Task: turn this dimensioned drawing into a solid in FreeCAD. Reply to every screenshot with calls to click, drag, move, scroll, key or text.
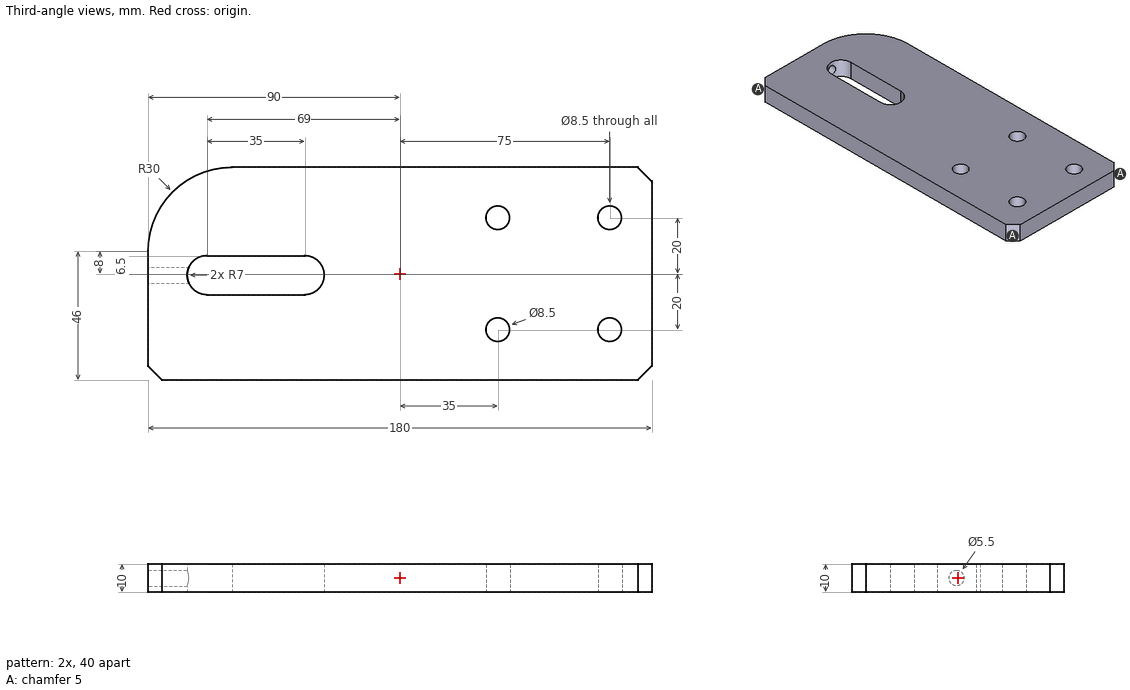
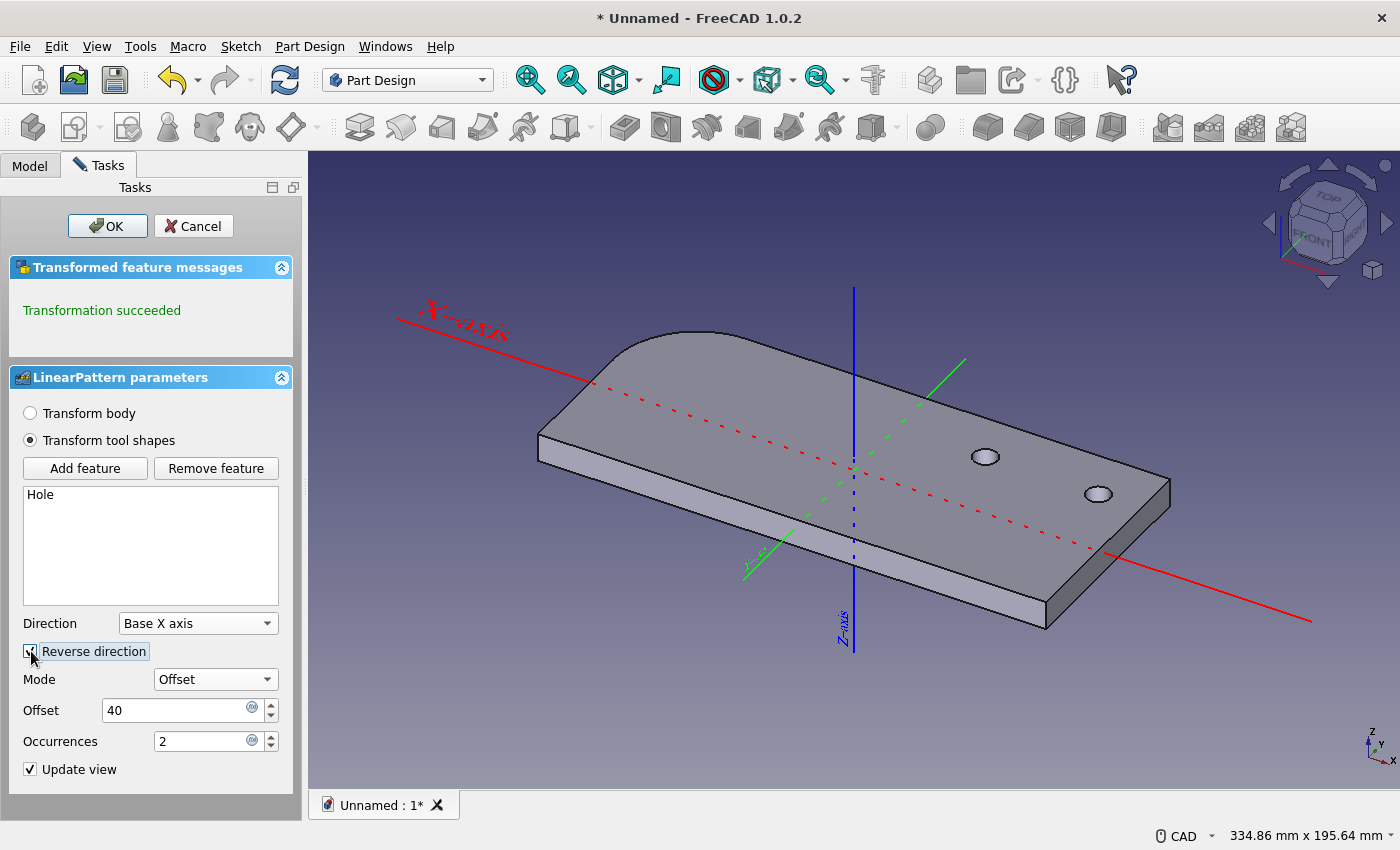
click(108, 226)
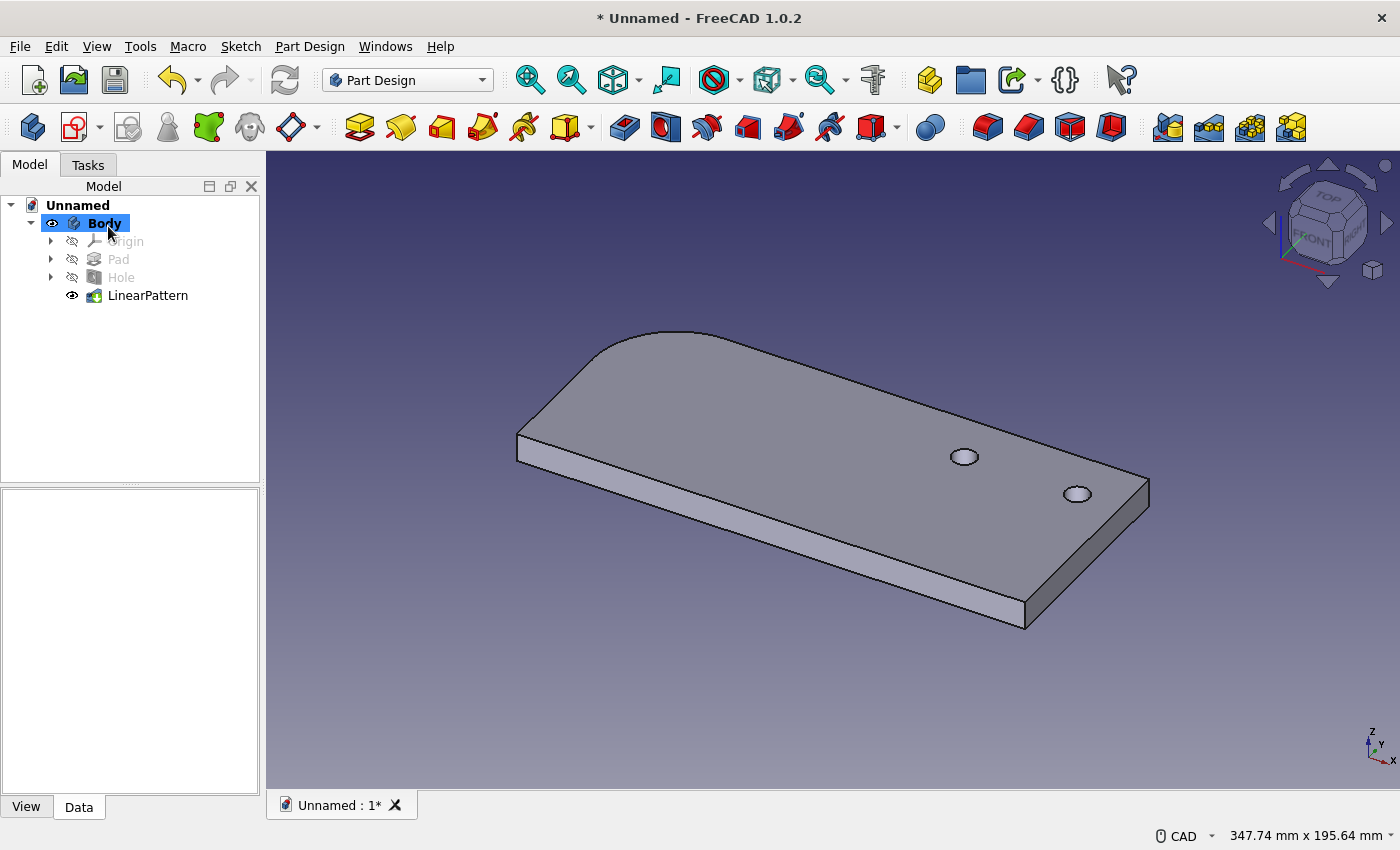
click(117, 277)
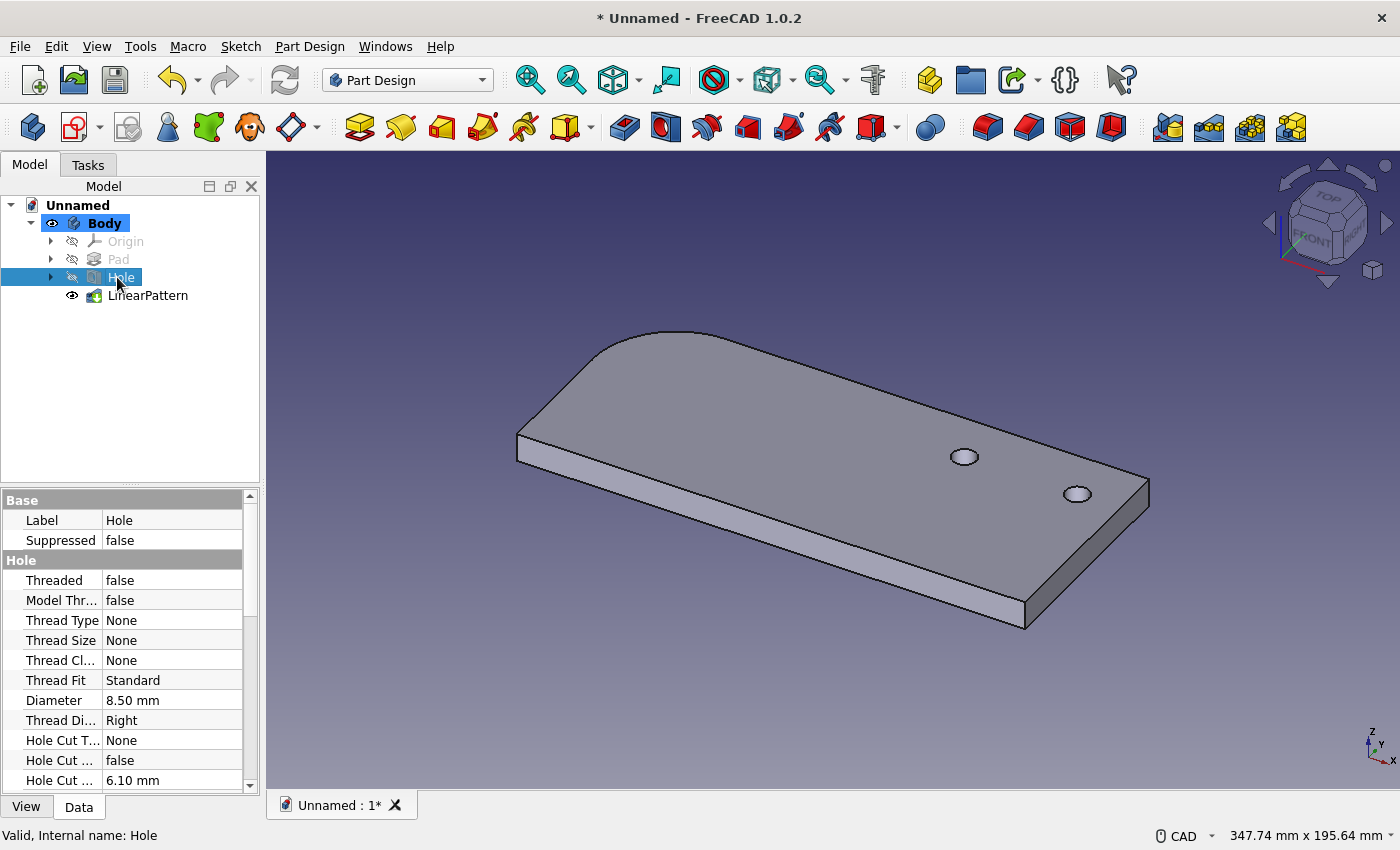
click(1168, 128)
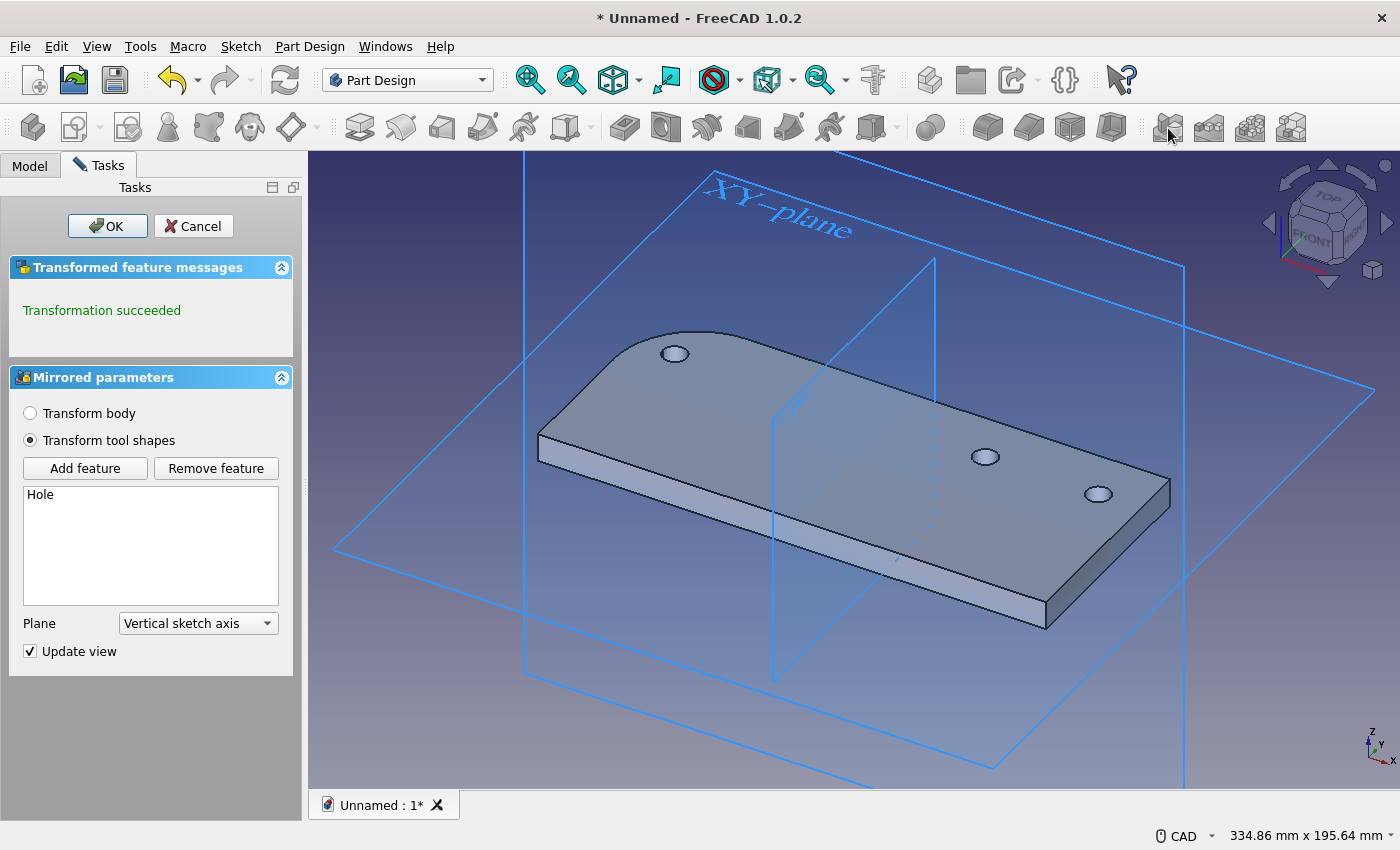
click(199, 624)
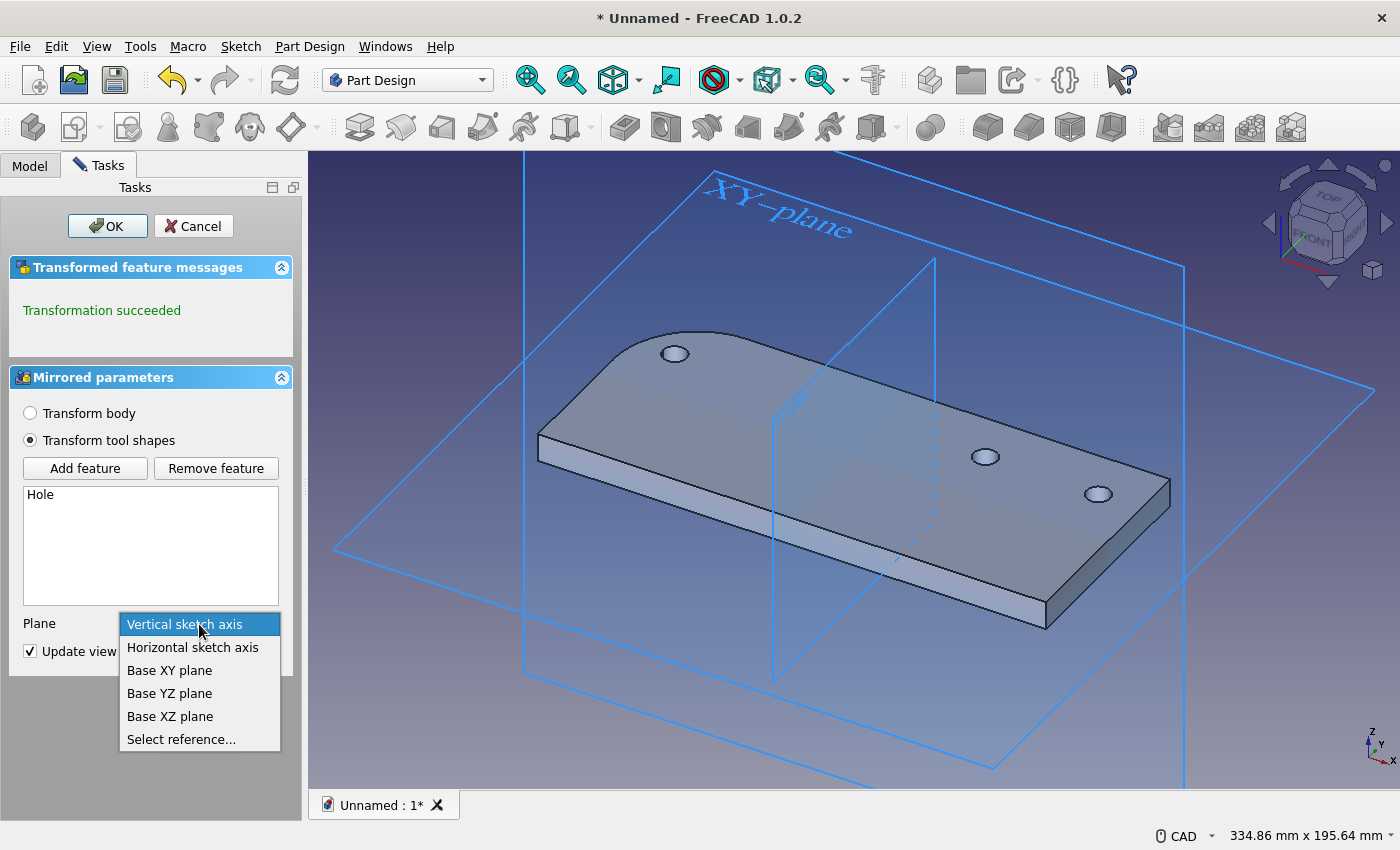
click(198, 716)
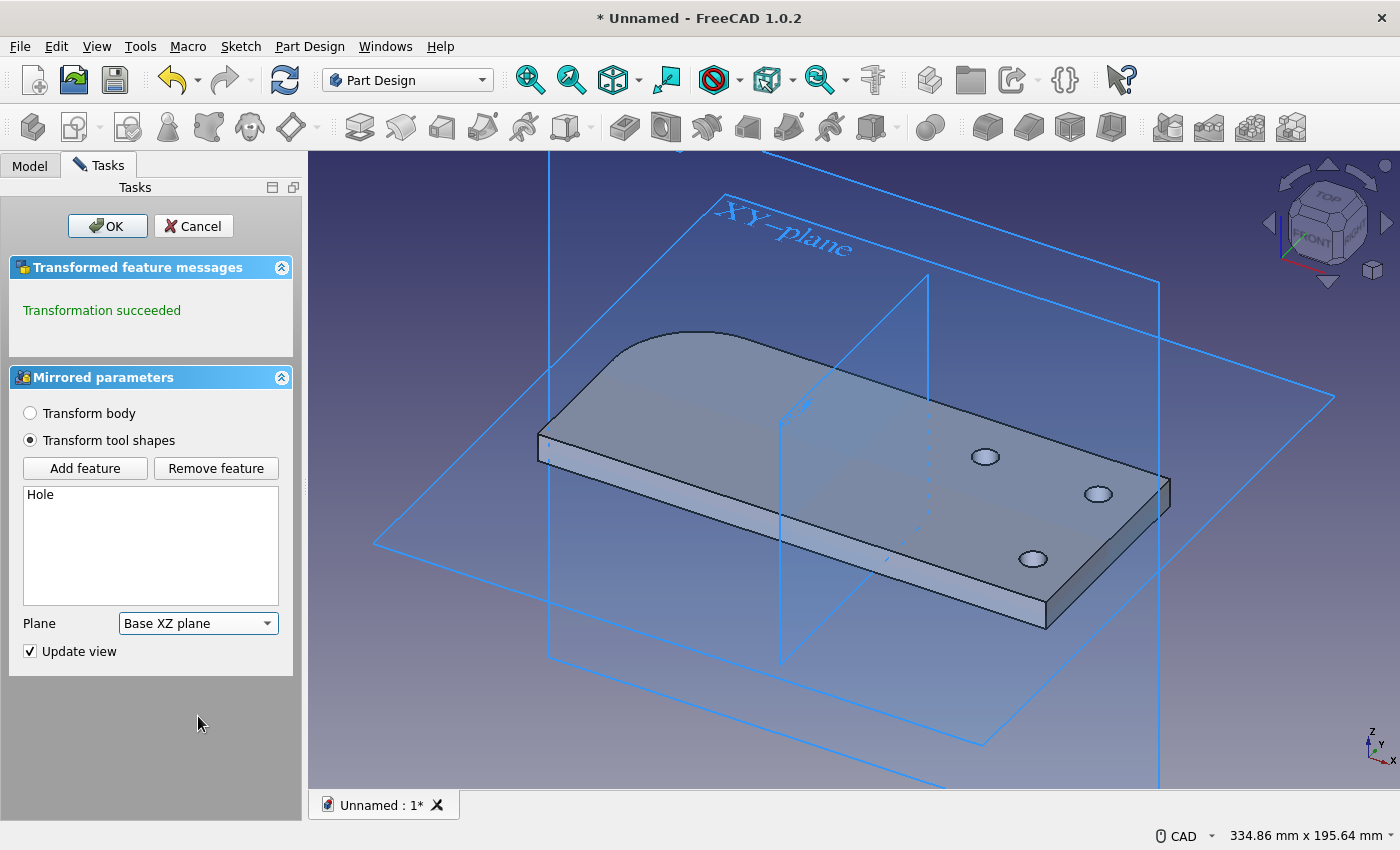
click(108, 226)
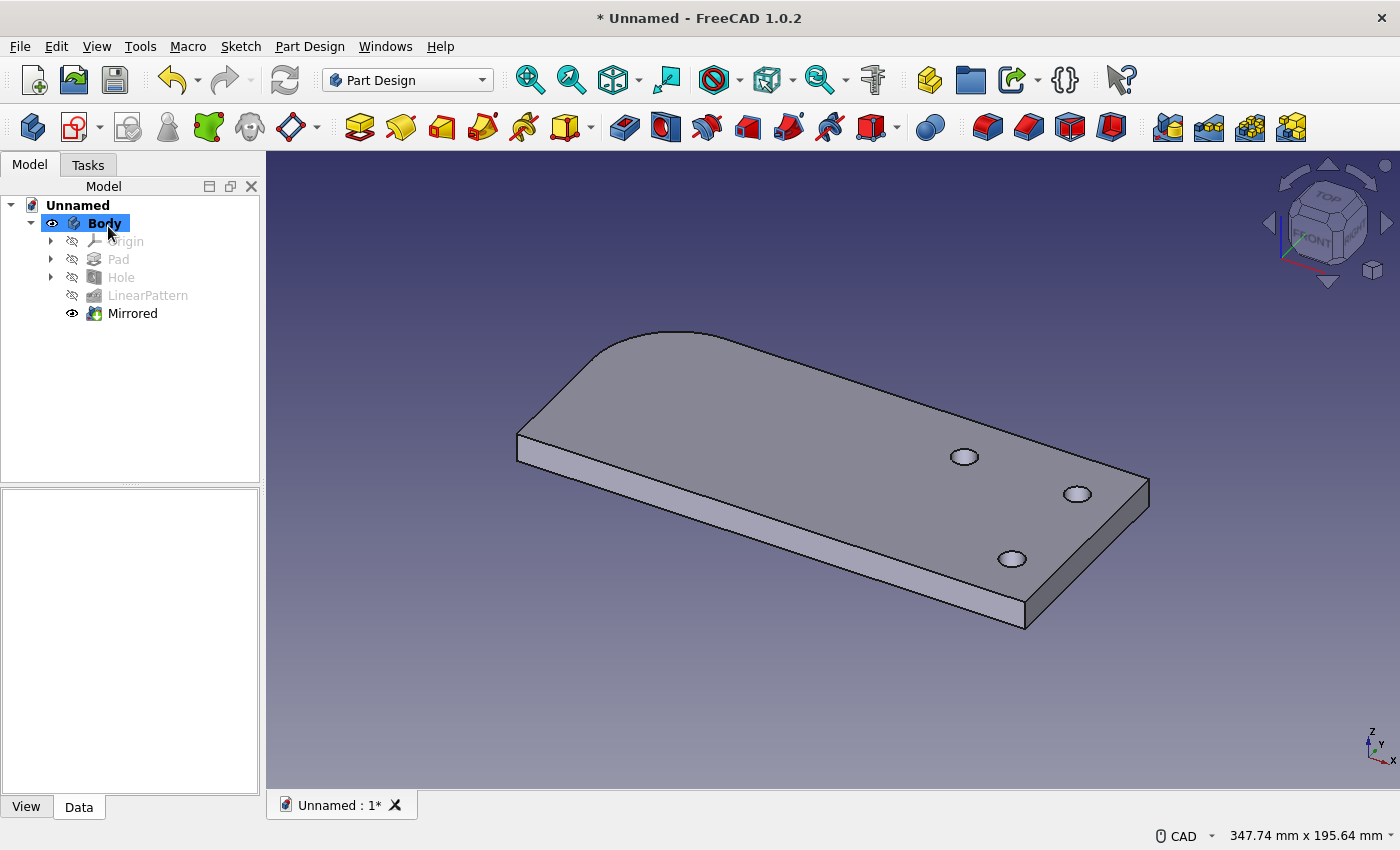
click(760, 432)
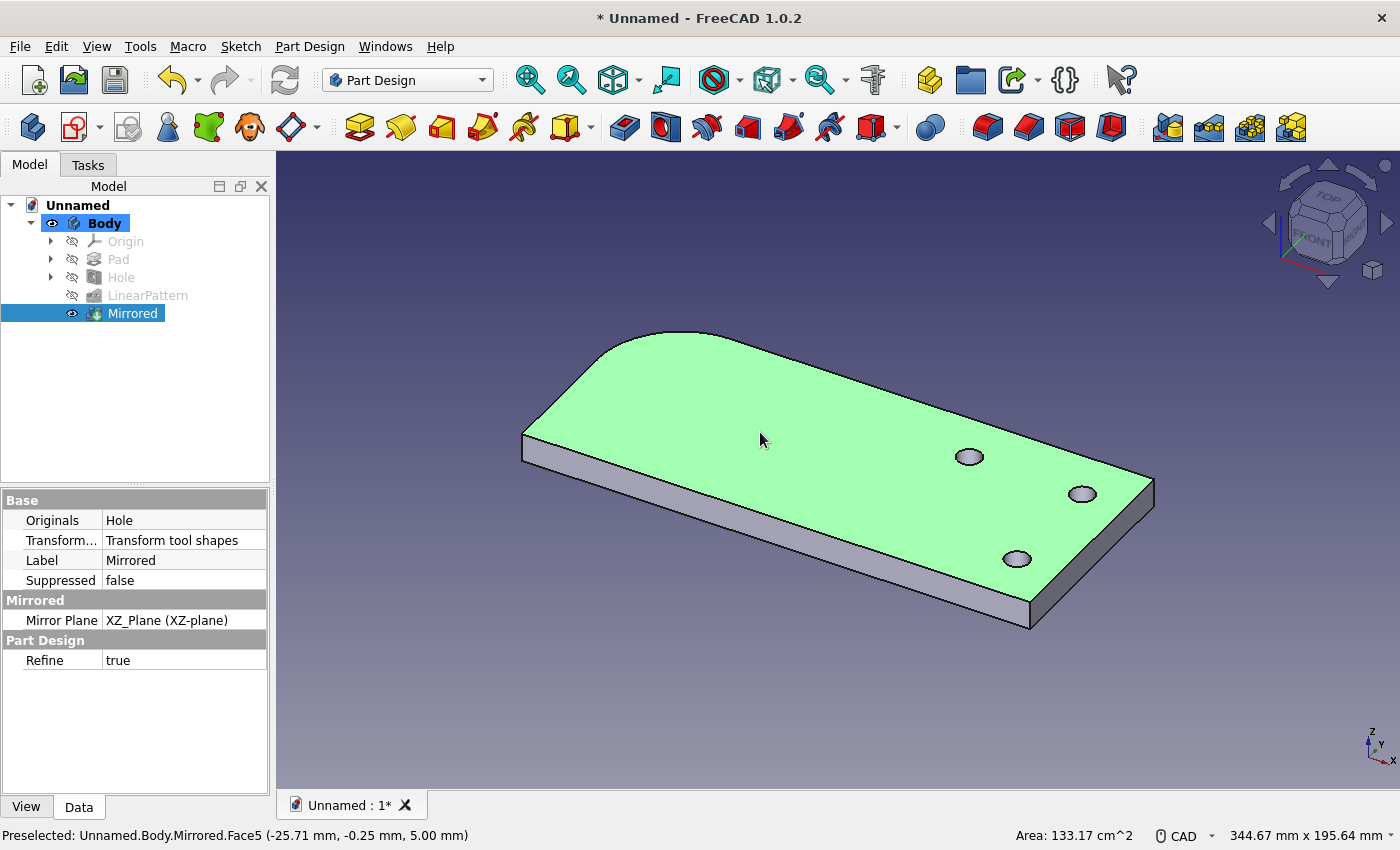
click(74, 128)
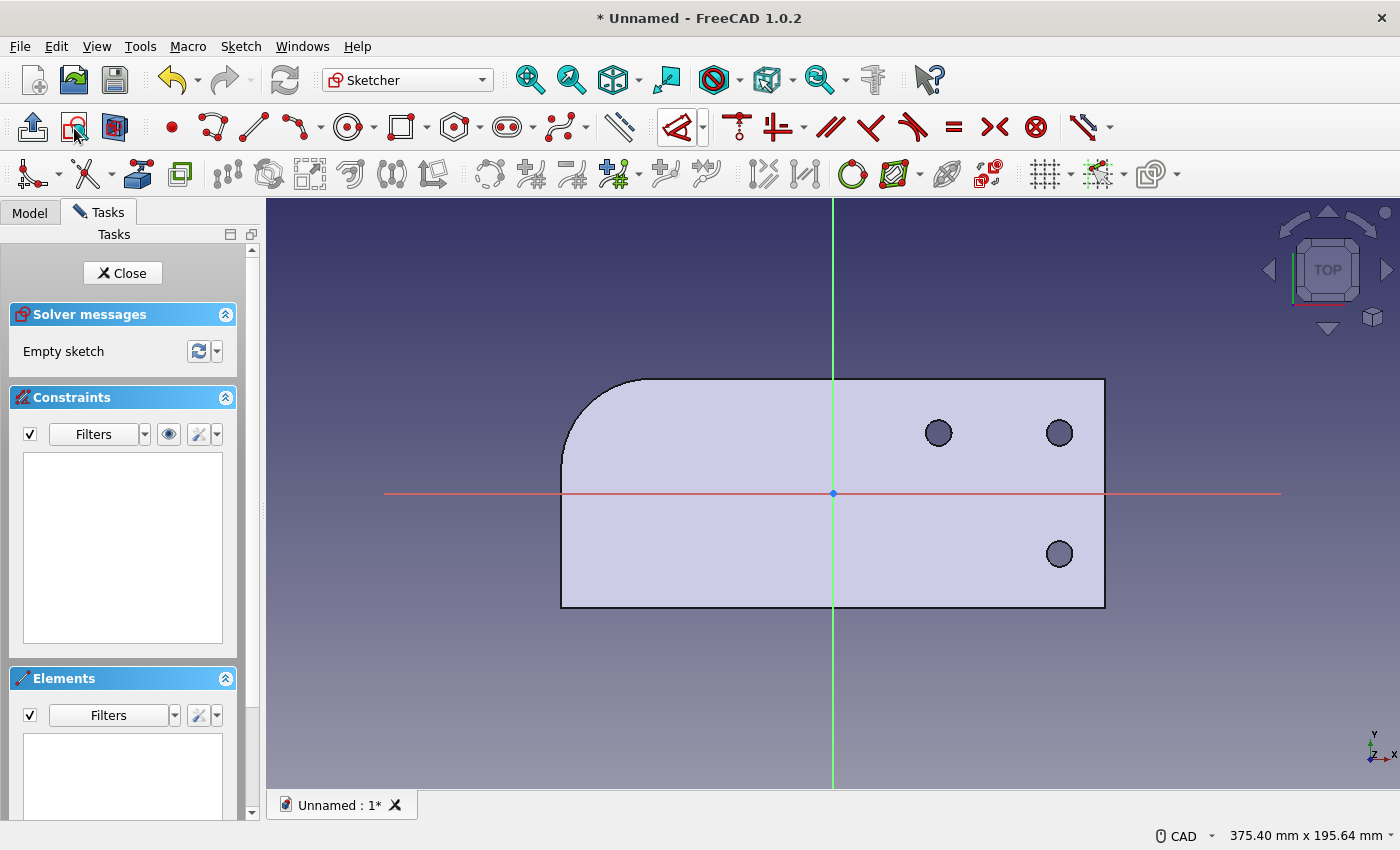
scroll(953, 559, up, 13)